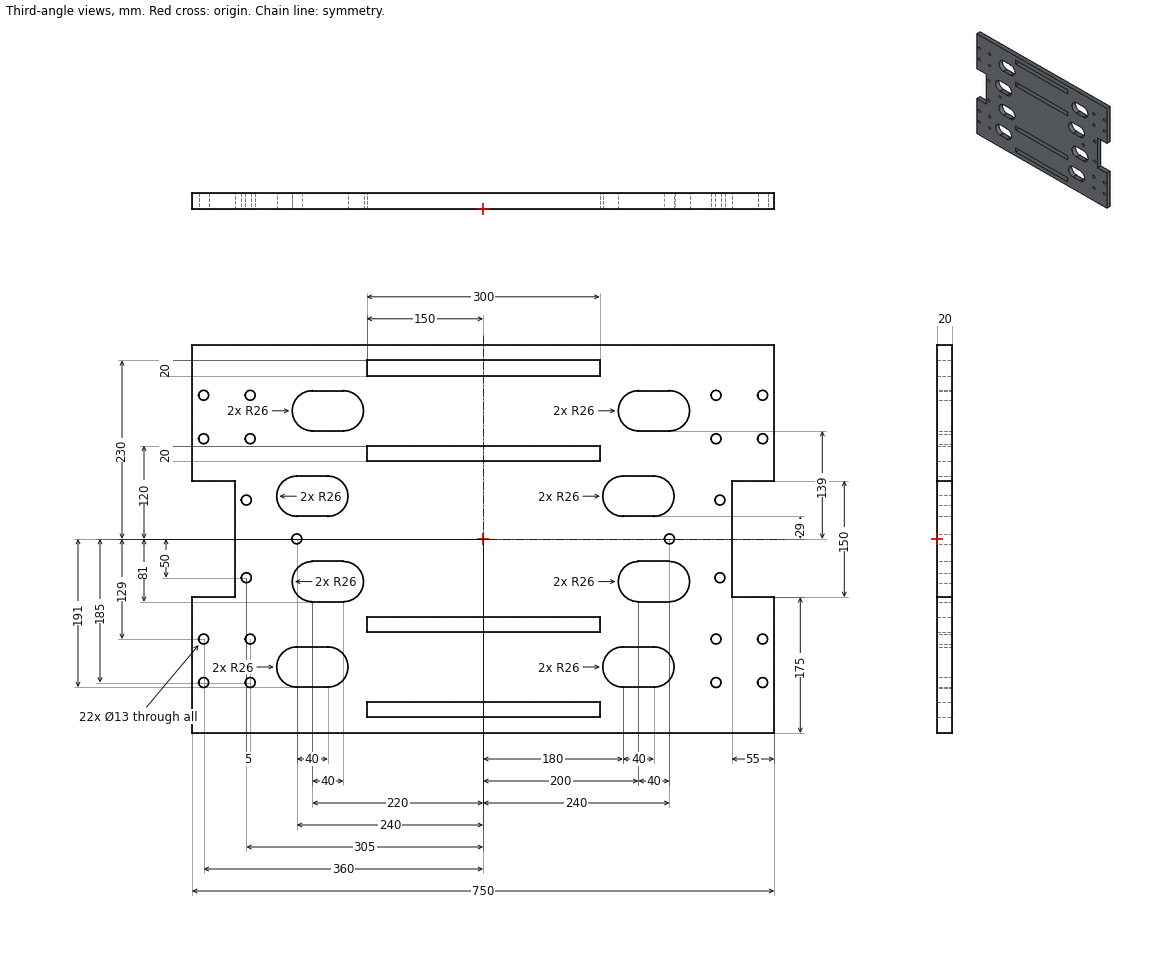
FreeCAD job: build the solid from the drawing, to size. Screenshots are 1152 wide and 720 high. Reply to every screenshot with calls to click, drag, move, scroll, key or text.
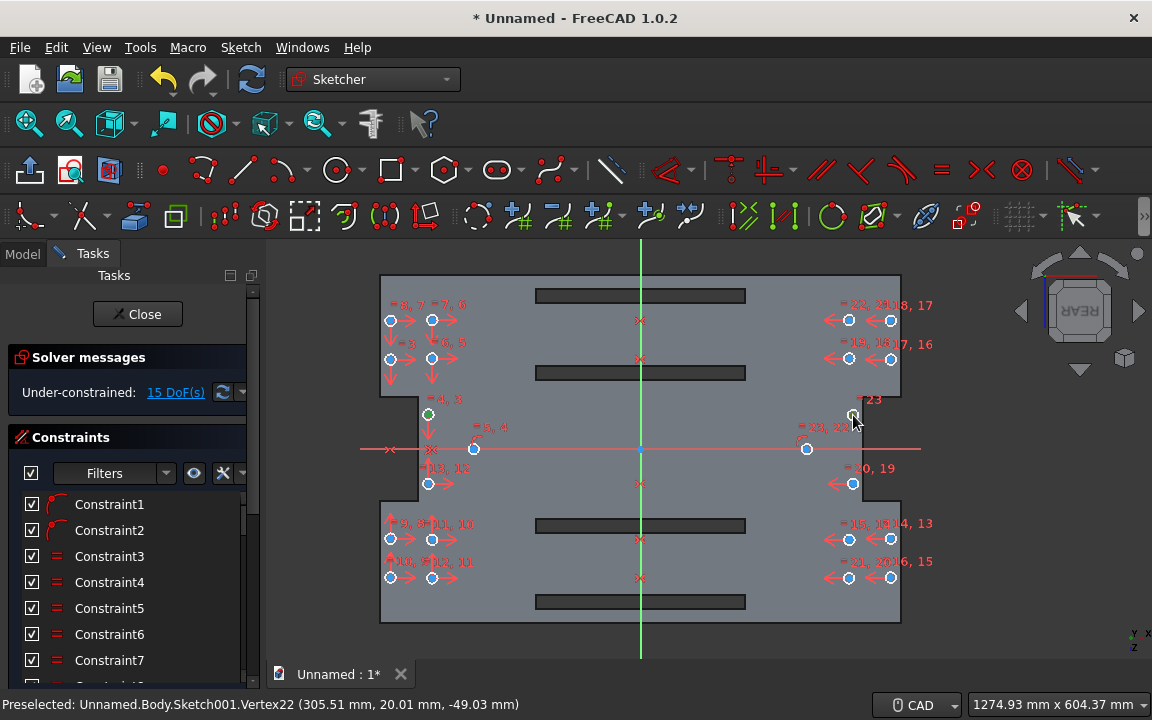
click(641, 605)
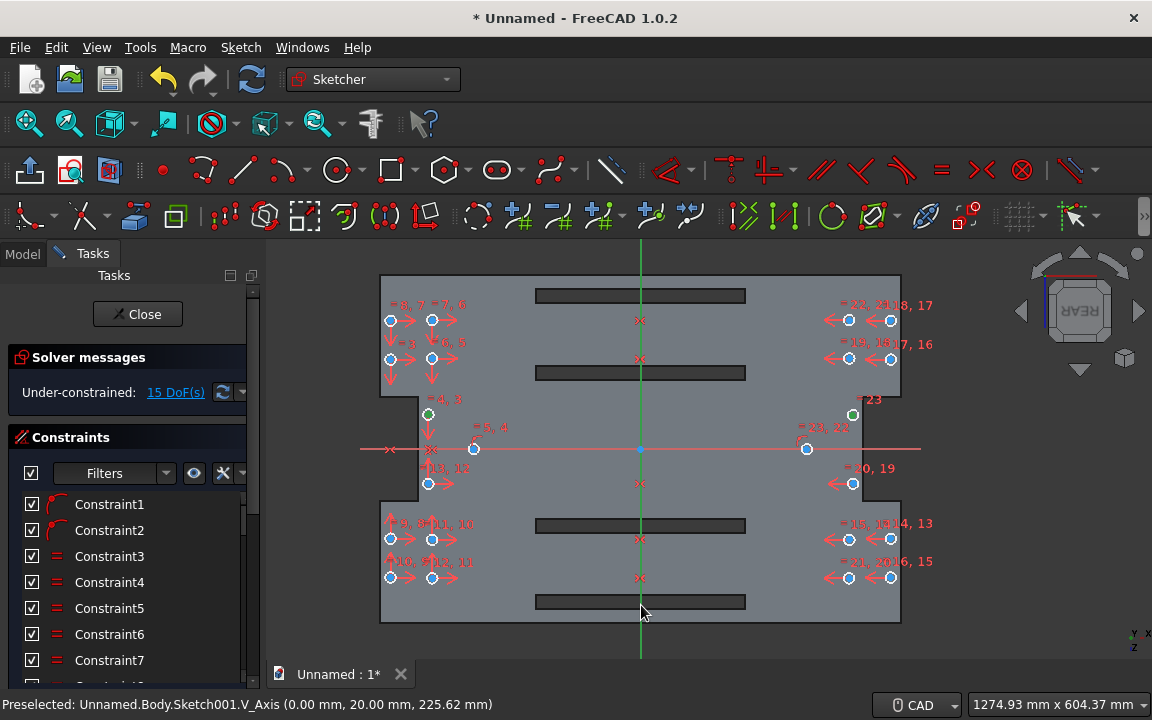
click(982, 170)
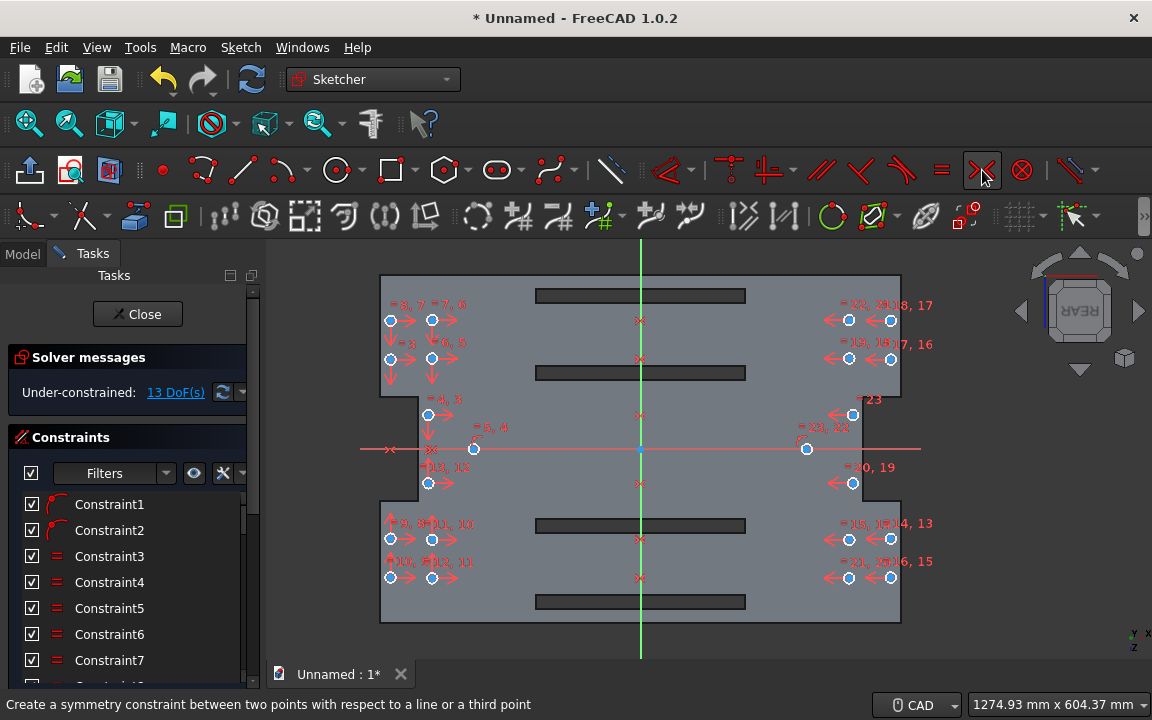
click(666, 170)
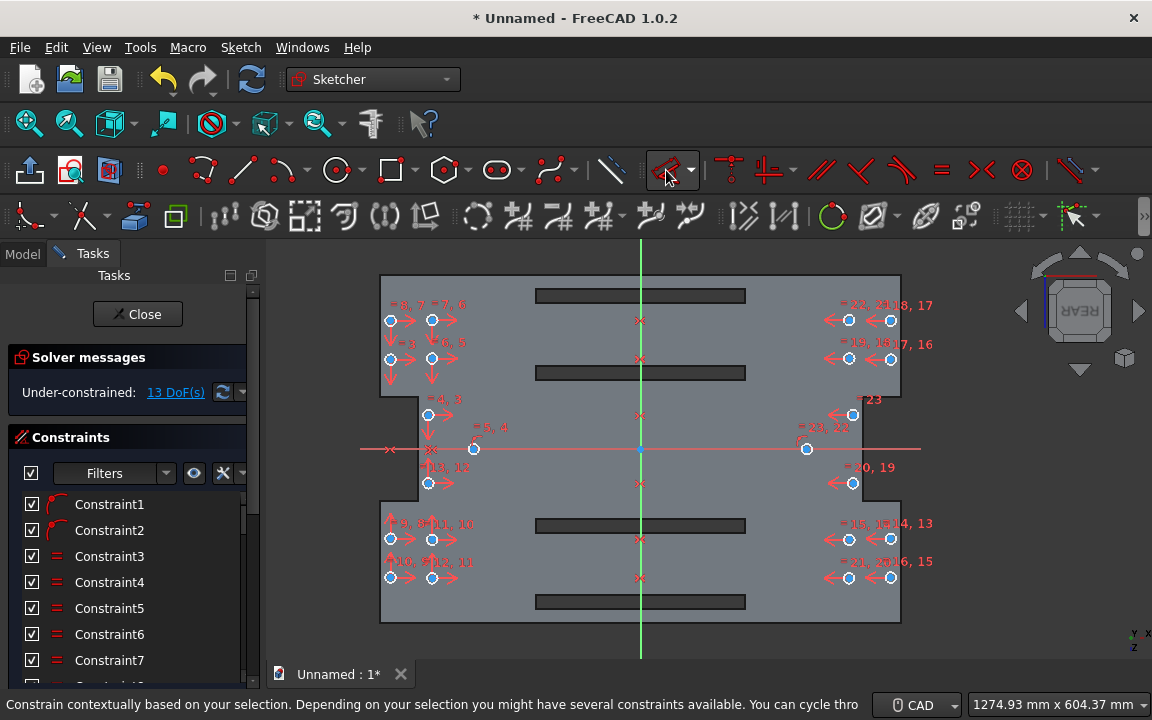
scroll(387, 356, up, 8)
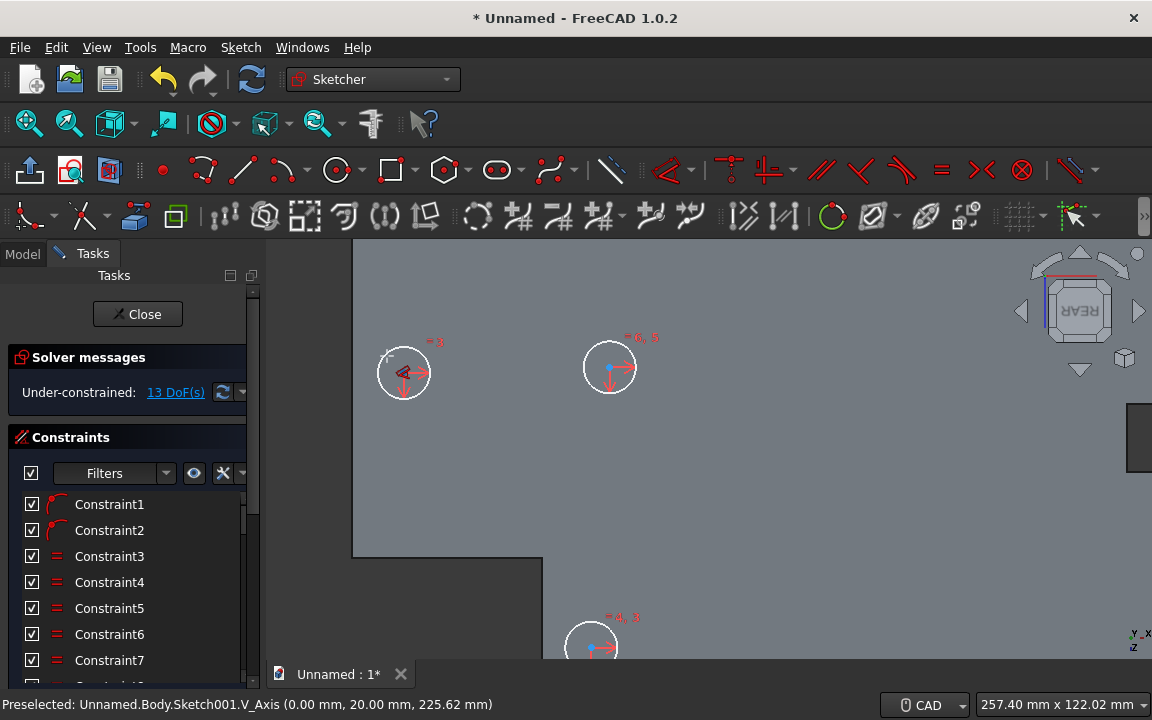
click(386, 355)
click(363, 332)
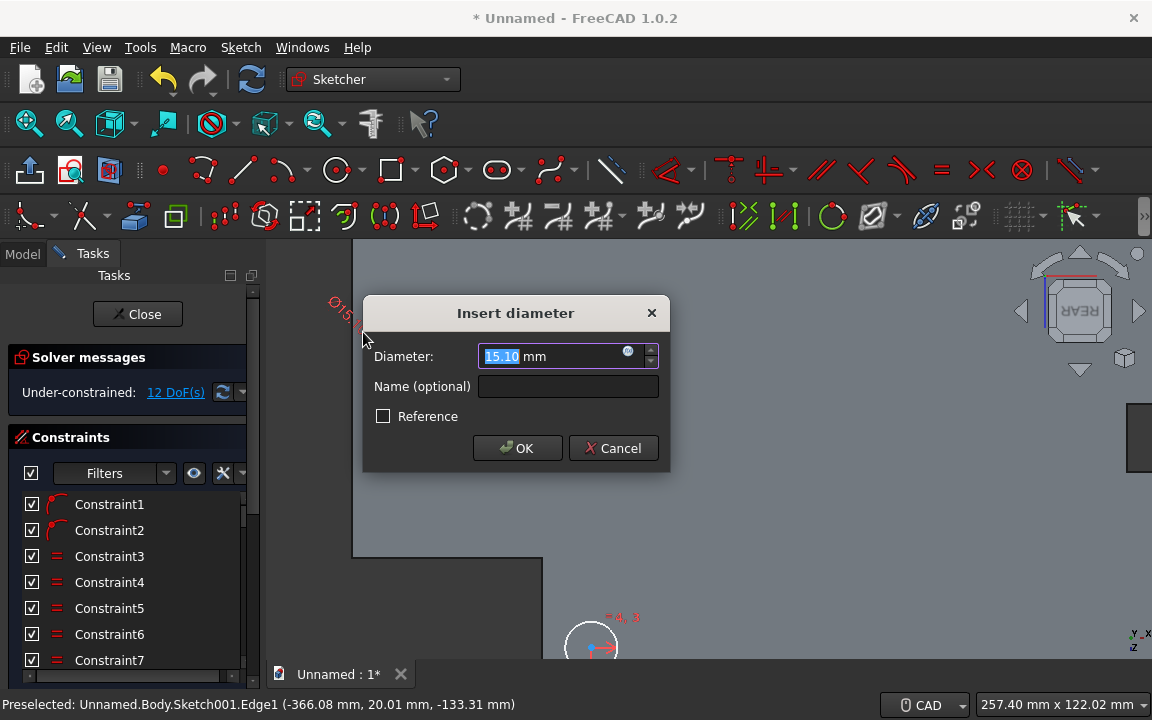
text(13)
key(Return)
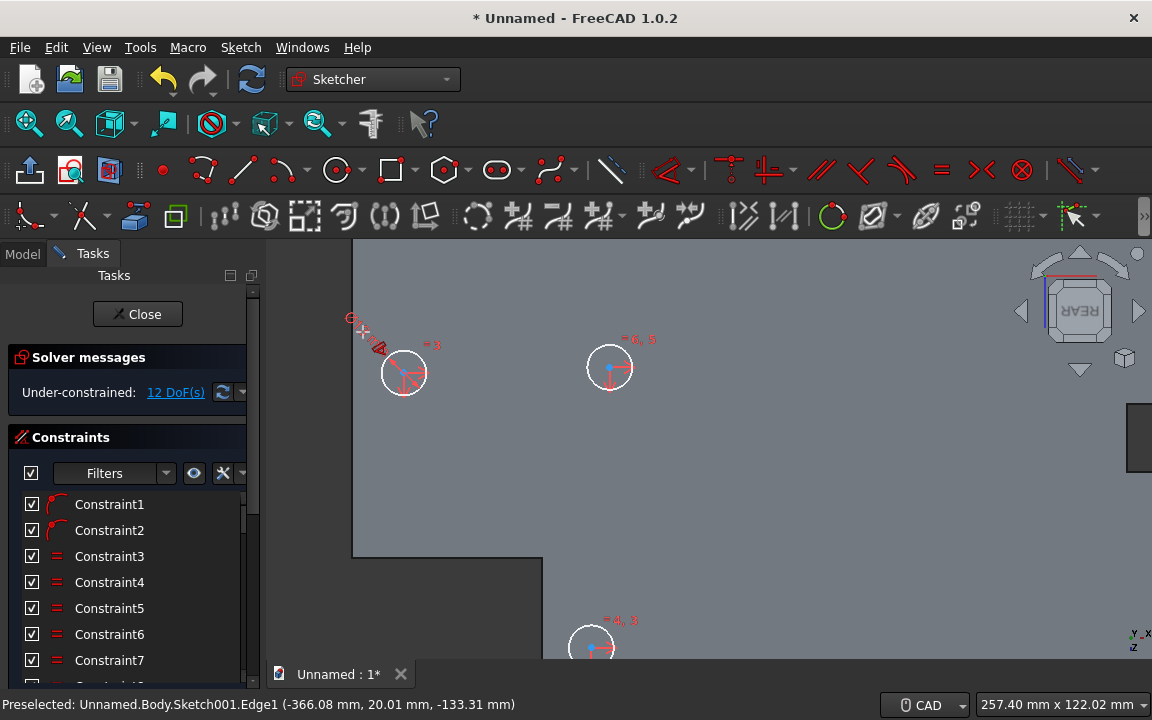
scroll(387, 356, down, 8)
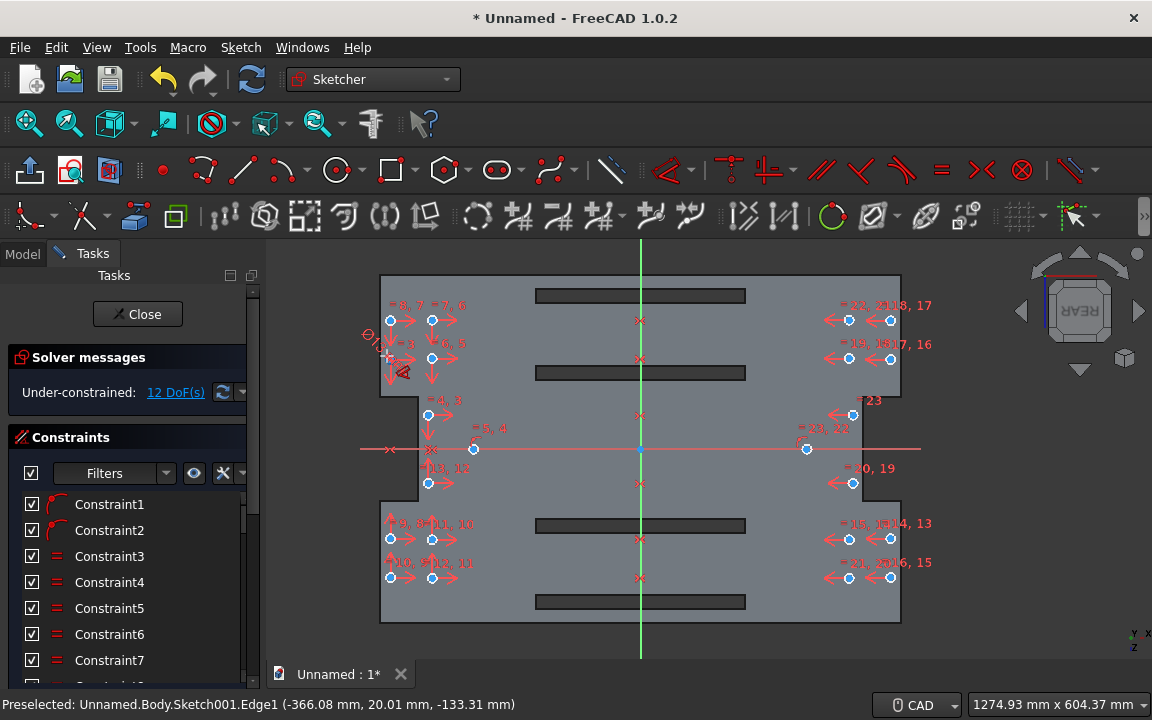
click(428, 415)
click(394, 432)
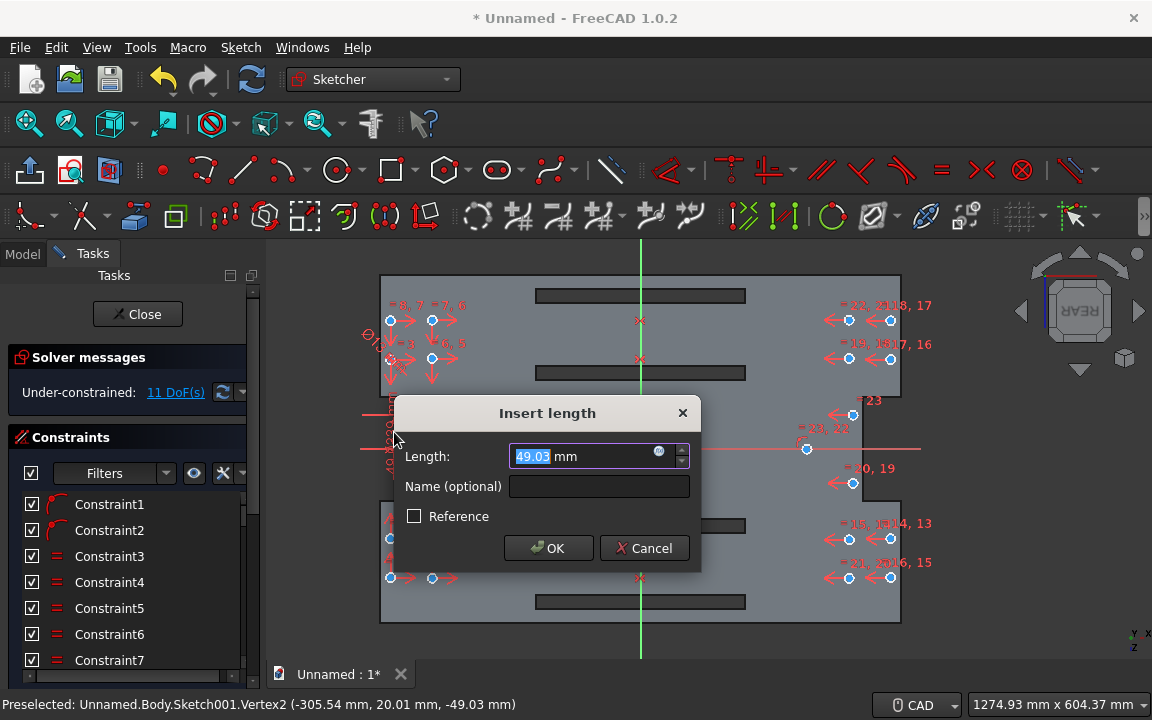
text(50)
key(Return)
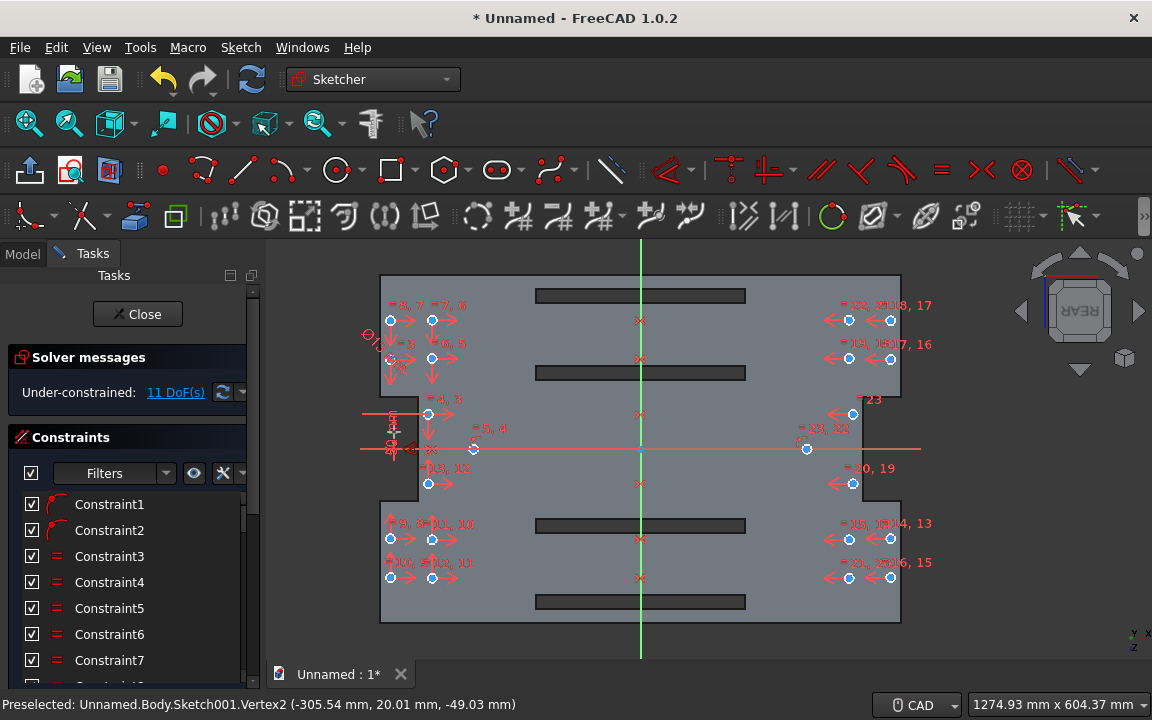
scroll(428, 414, up, 13)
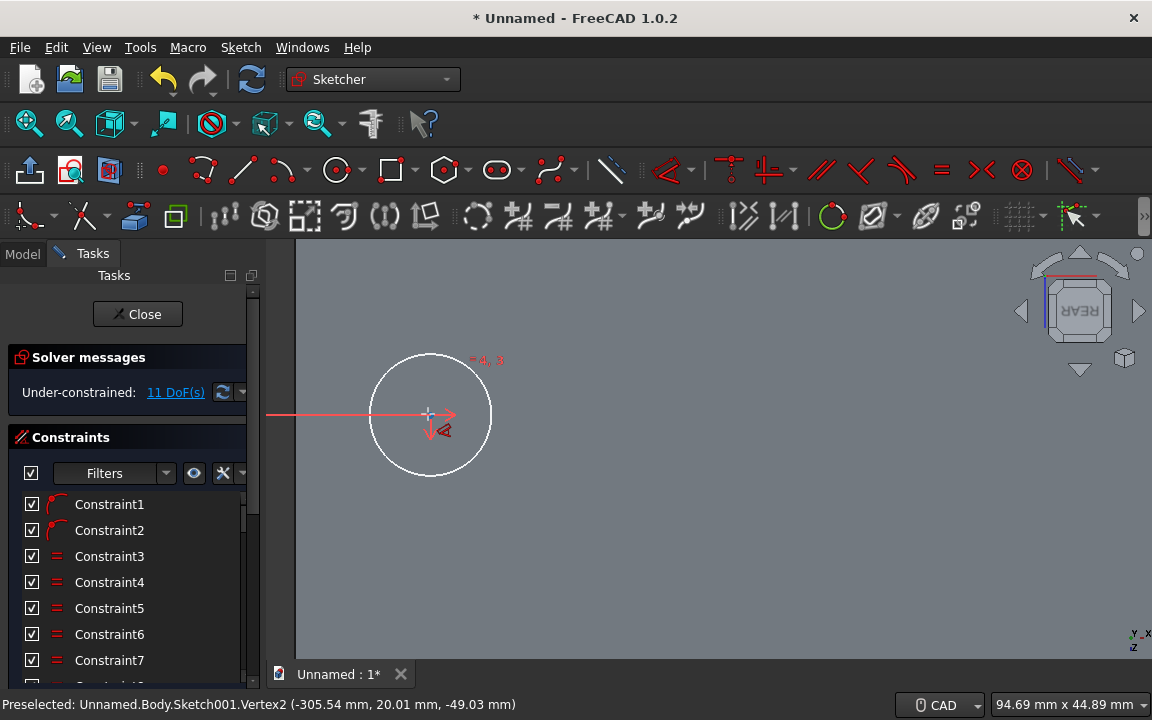
click(431, 415)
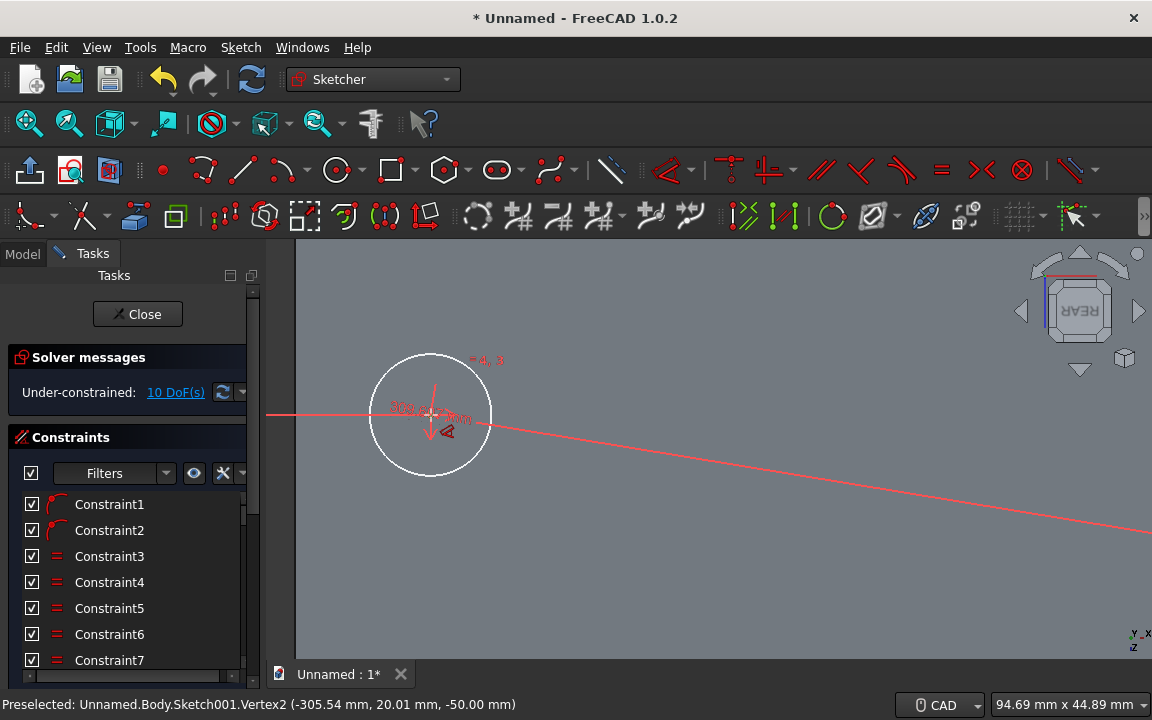
scroll(428, 414, down, 13)